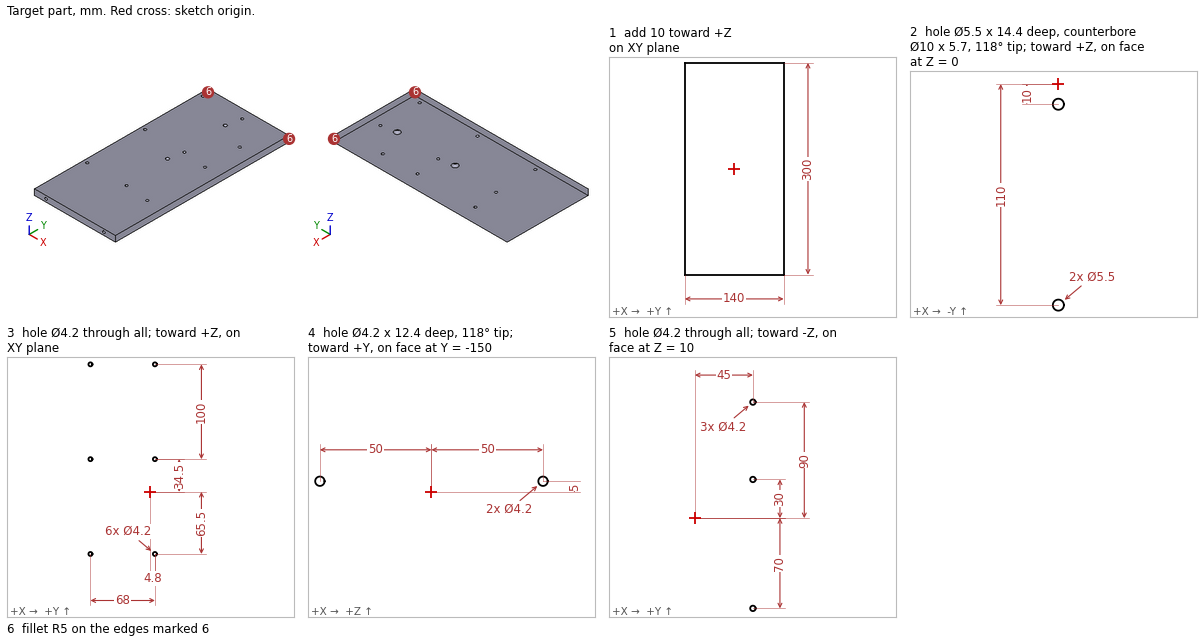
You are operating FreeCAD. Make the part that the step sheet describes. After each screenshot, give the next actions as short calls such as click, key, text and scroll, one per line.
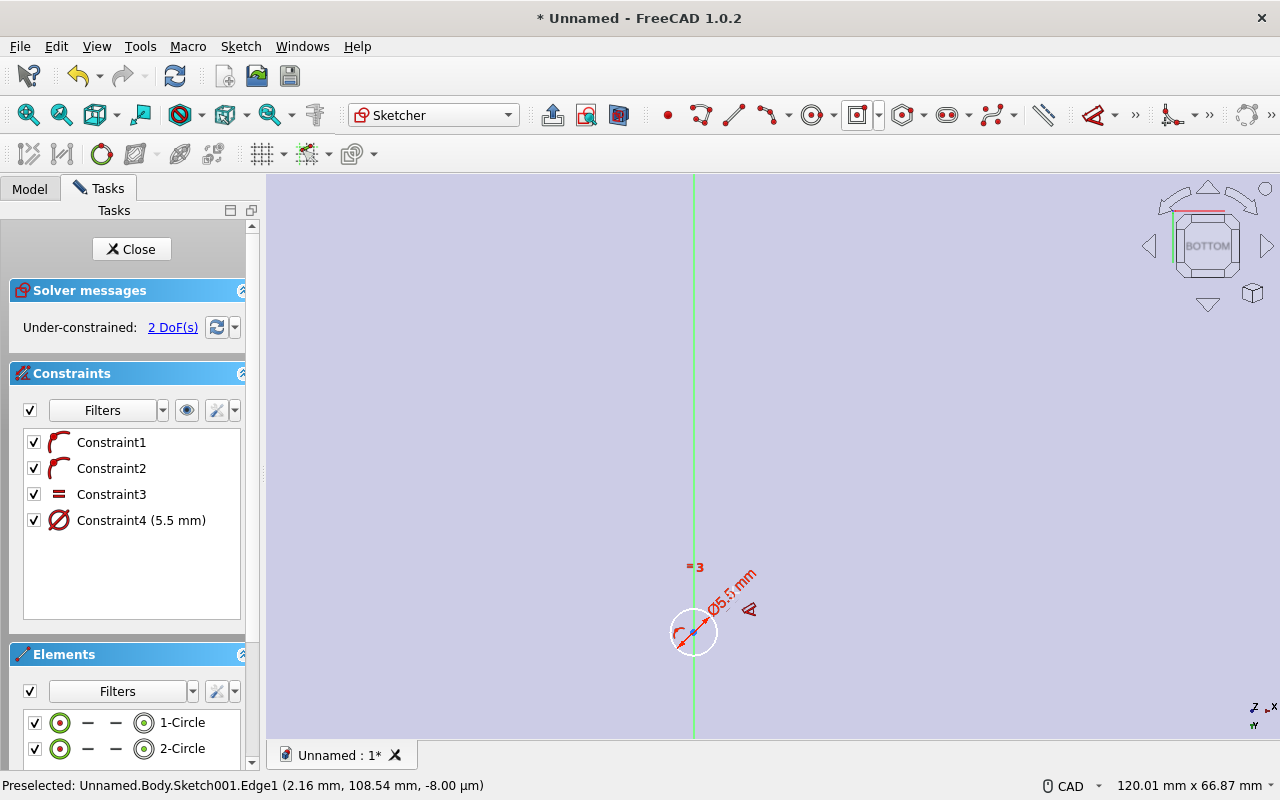
scroll(711, 618, down, 5)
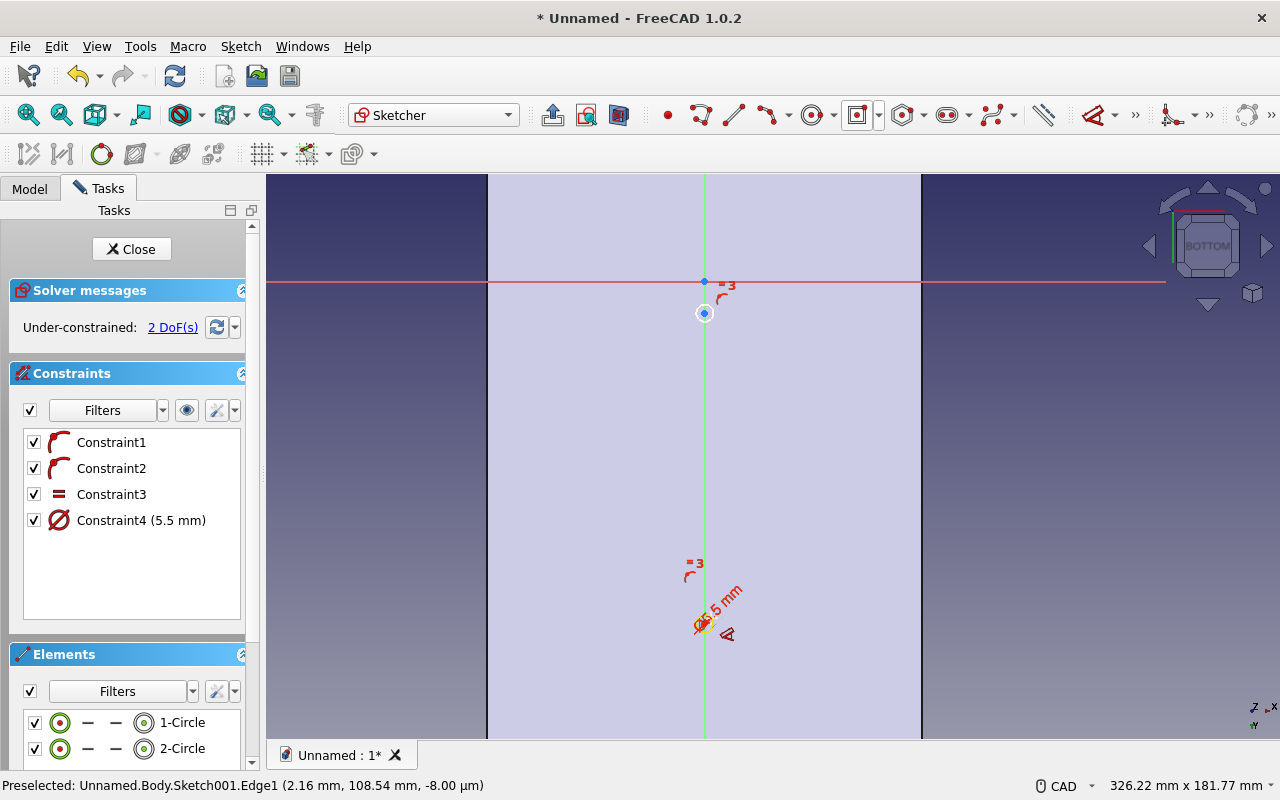
scroll(705, 313, up, 2)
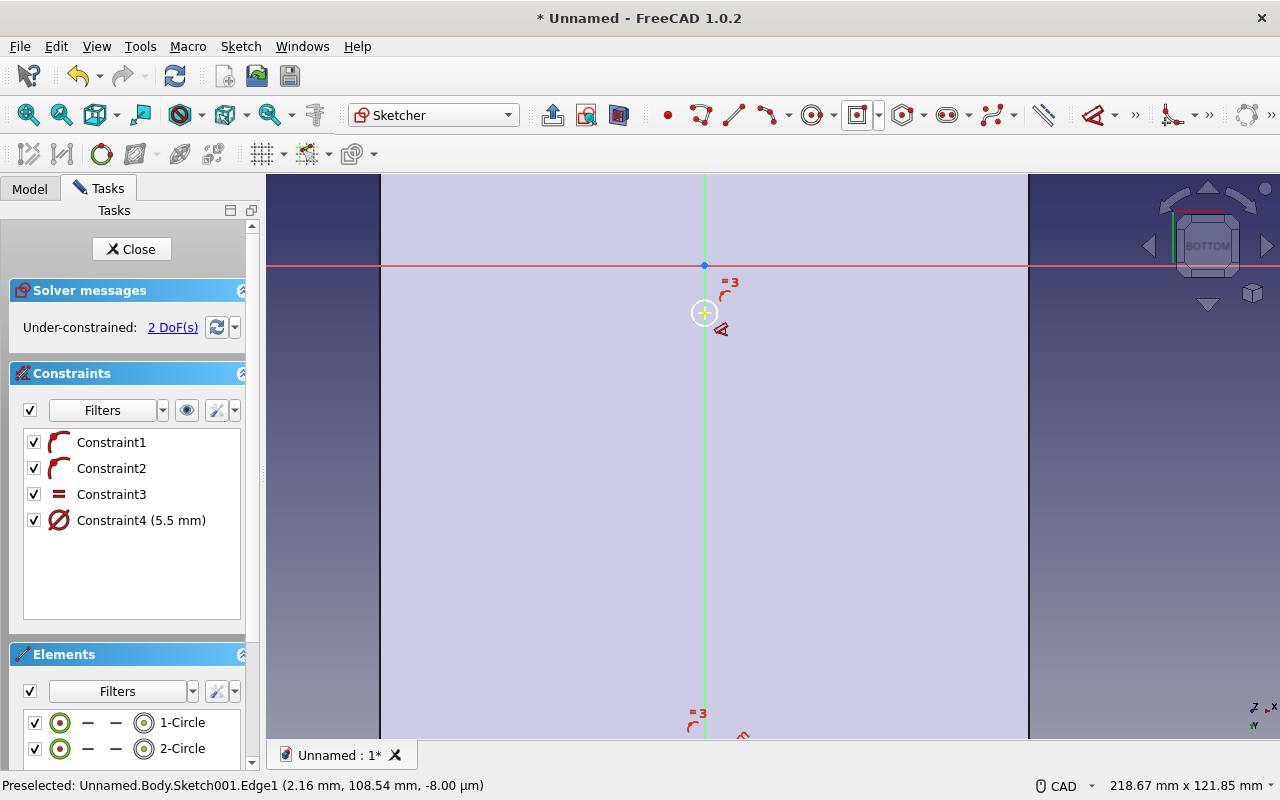
click(705, 313)
click(739, 290)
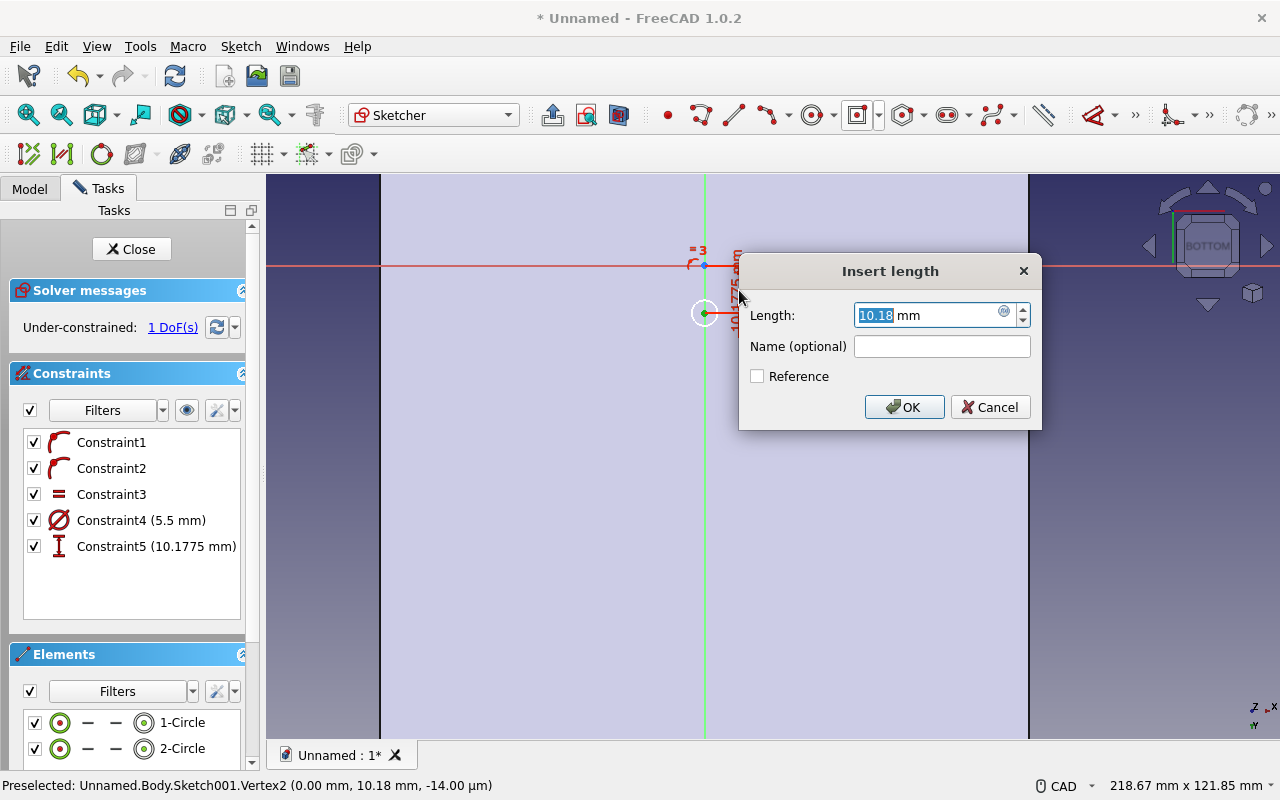
text(10)
key(Return)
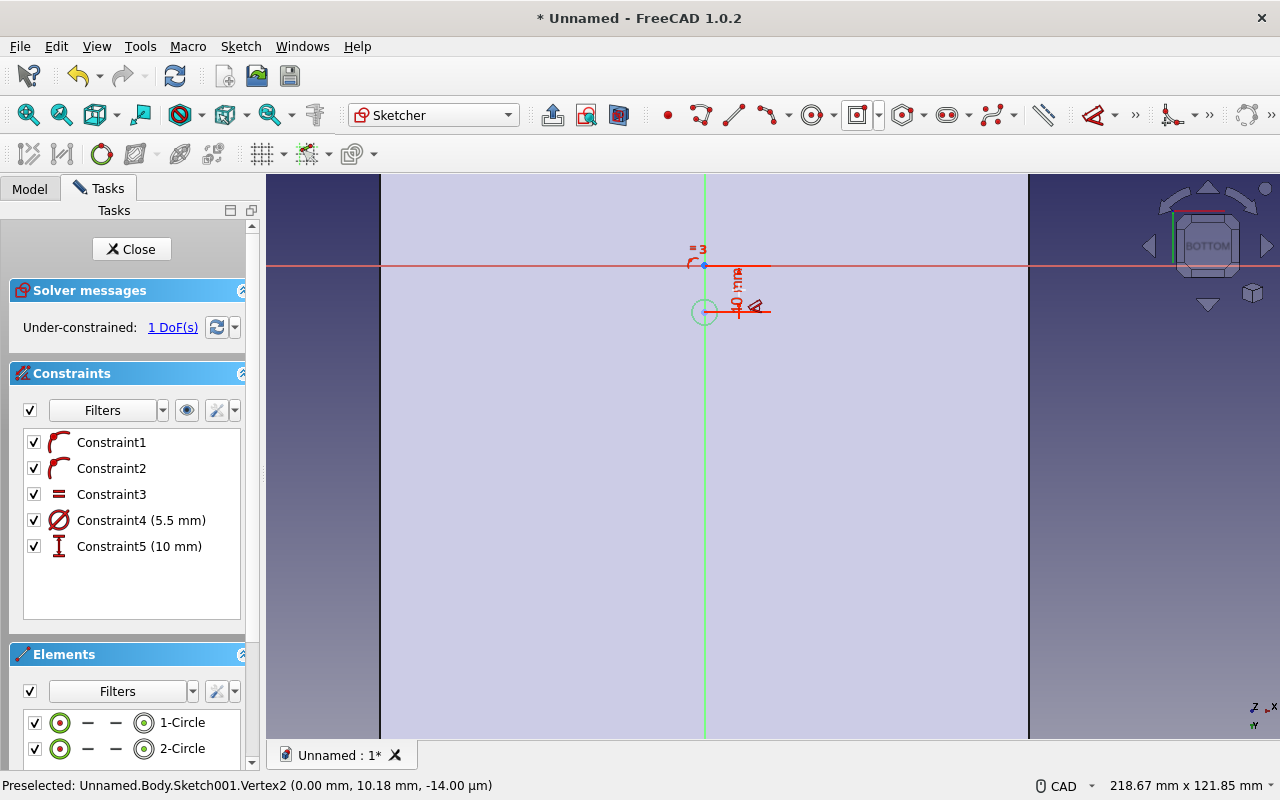
scroll(704, 312, down, 2)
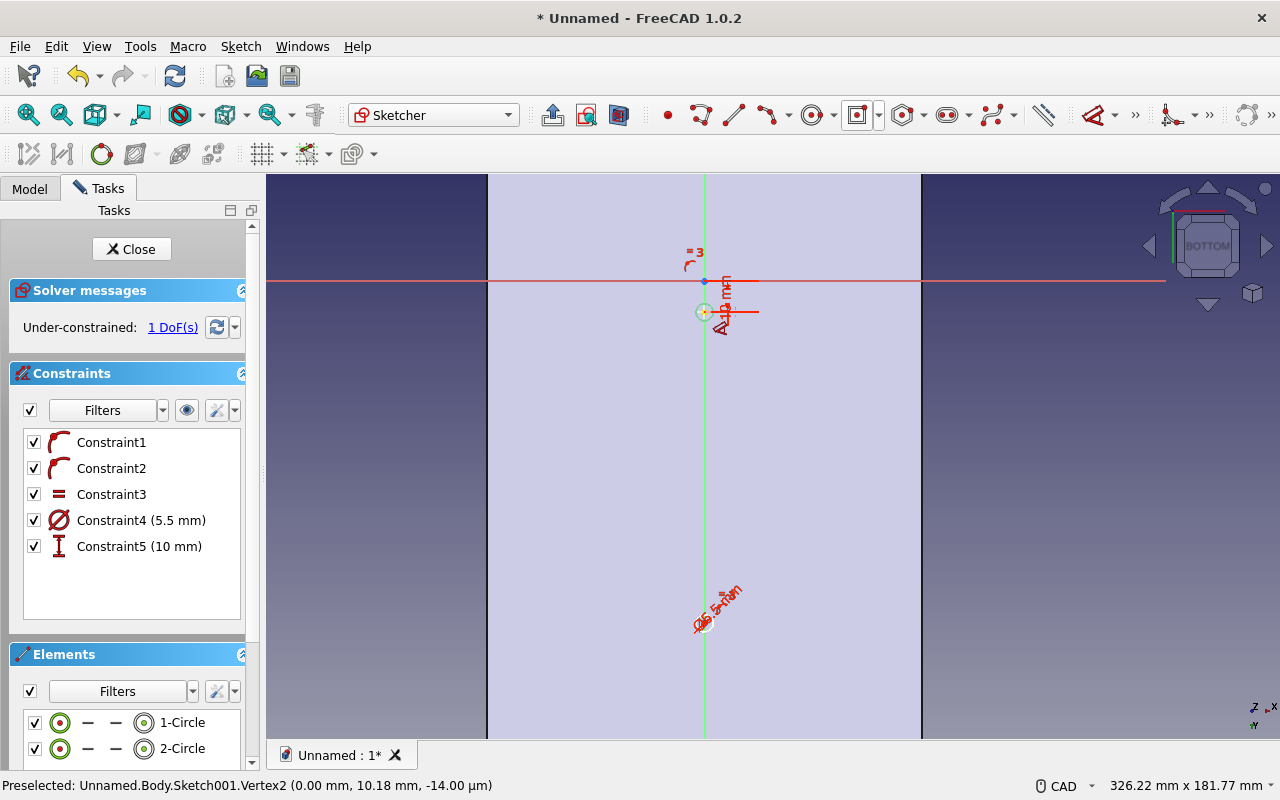
click(705, 623)
click(739, 452)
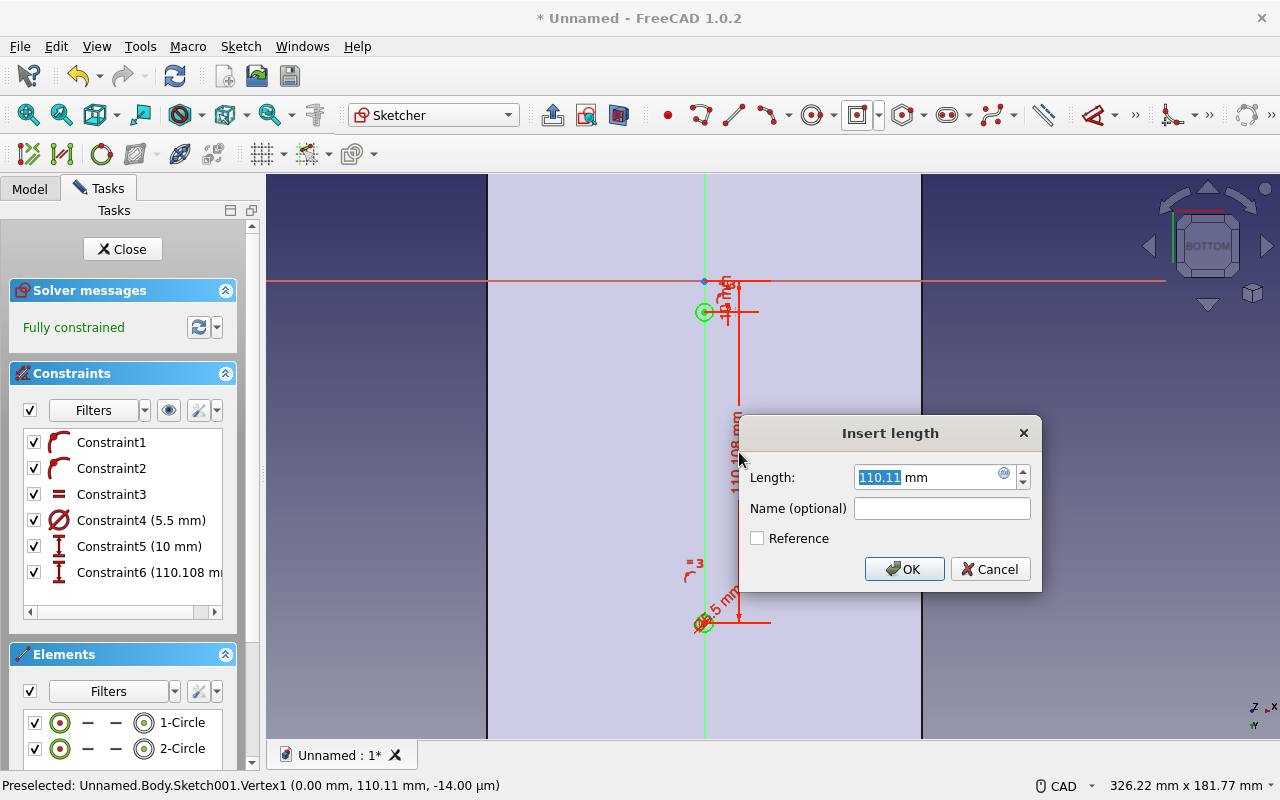
text(110)
key(Return)
key(Escape)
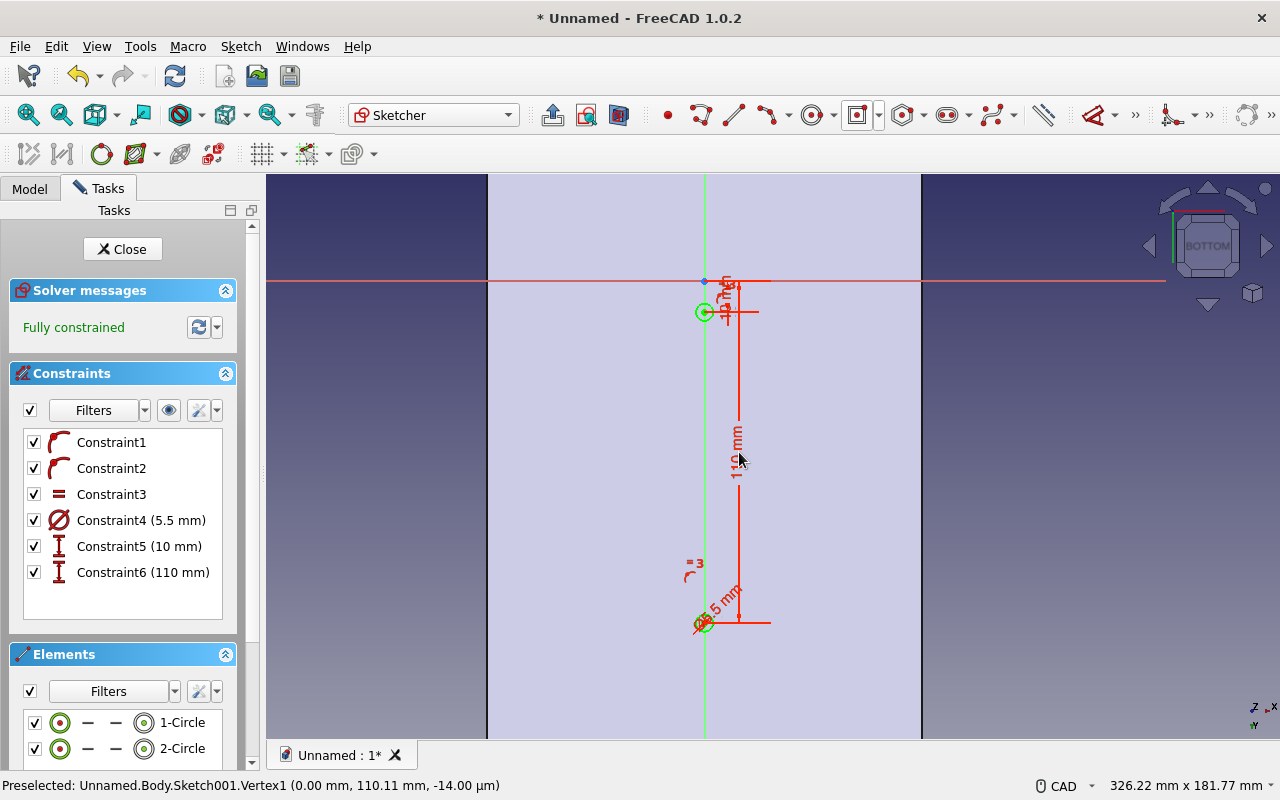
click(123, 249)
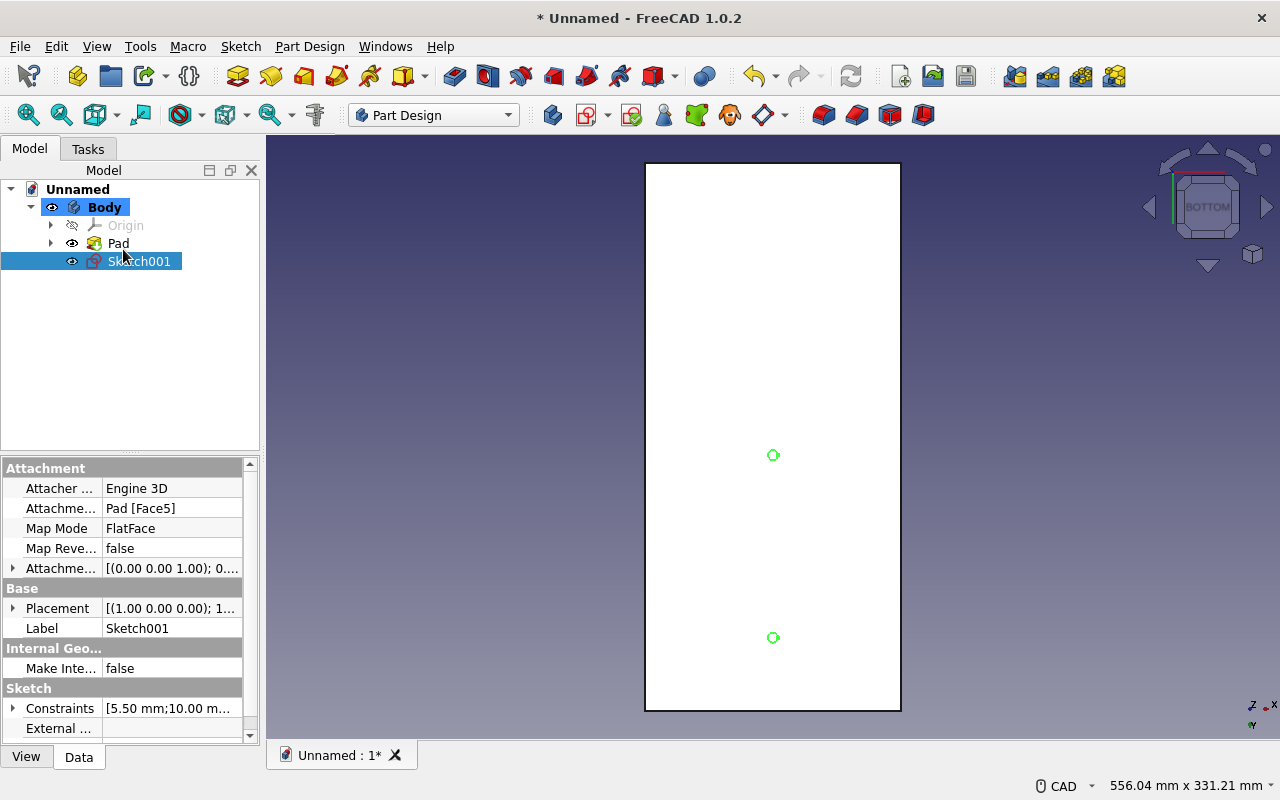
click(488, 76)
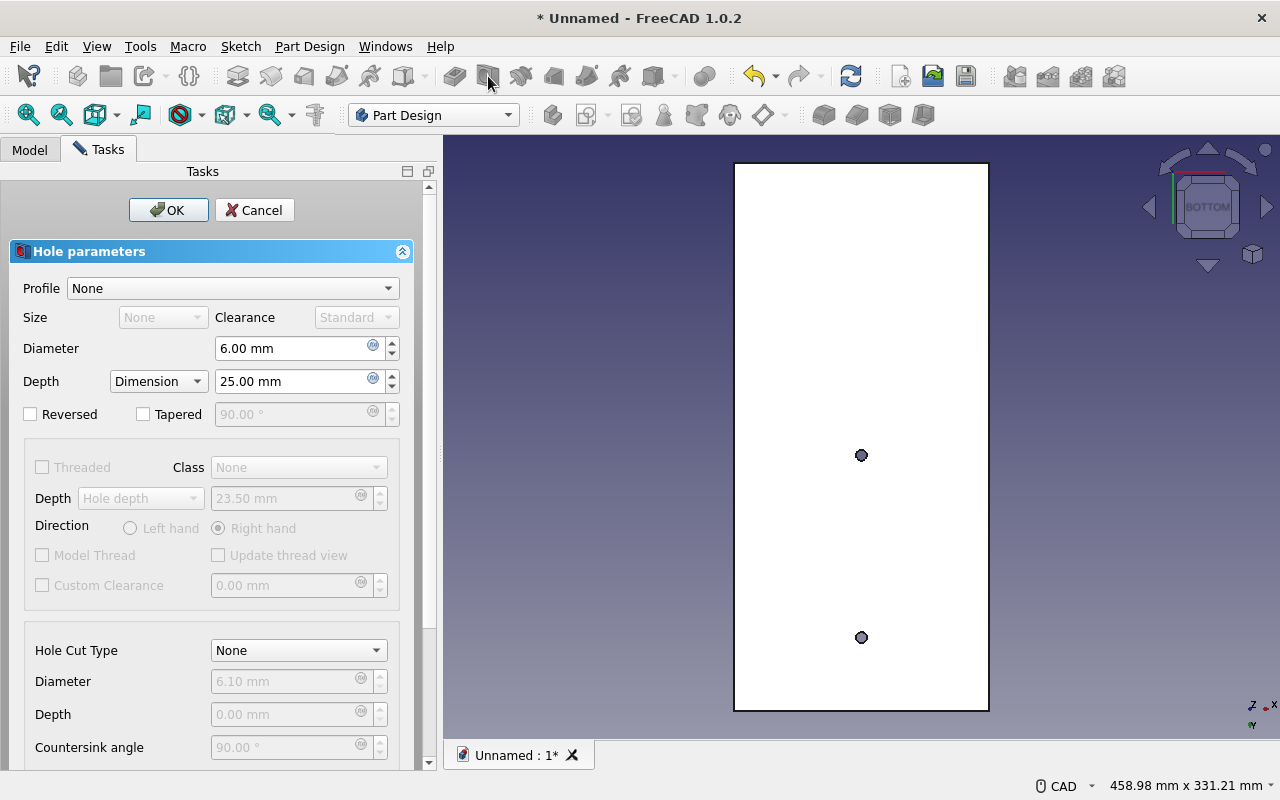
triple_click(300, 348)